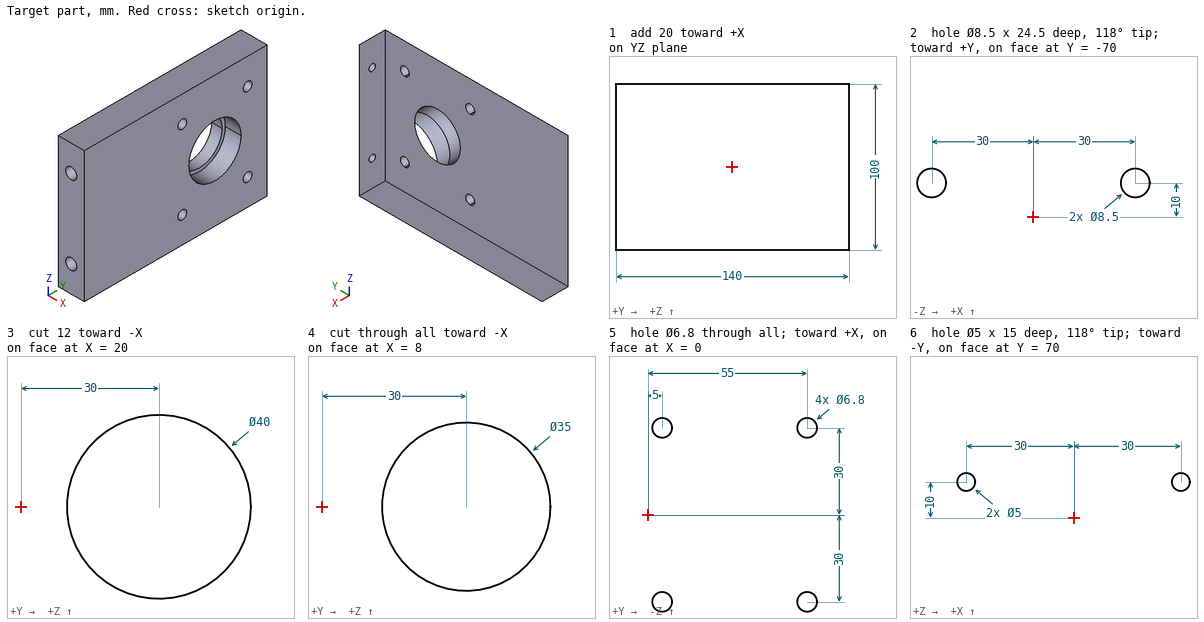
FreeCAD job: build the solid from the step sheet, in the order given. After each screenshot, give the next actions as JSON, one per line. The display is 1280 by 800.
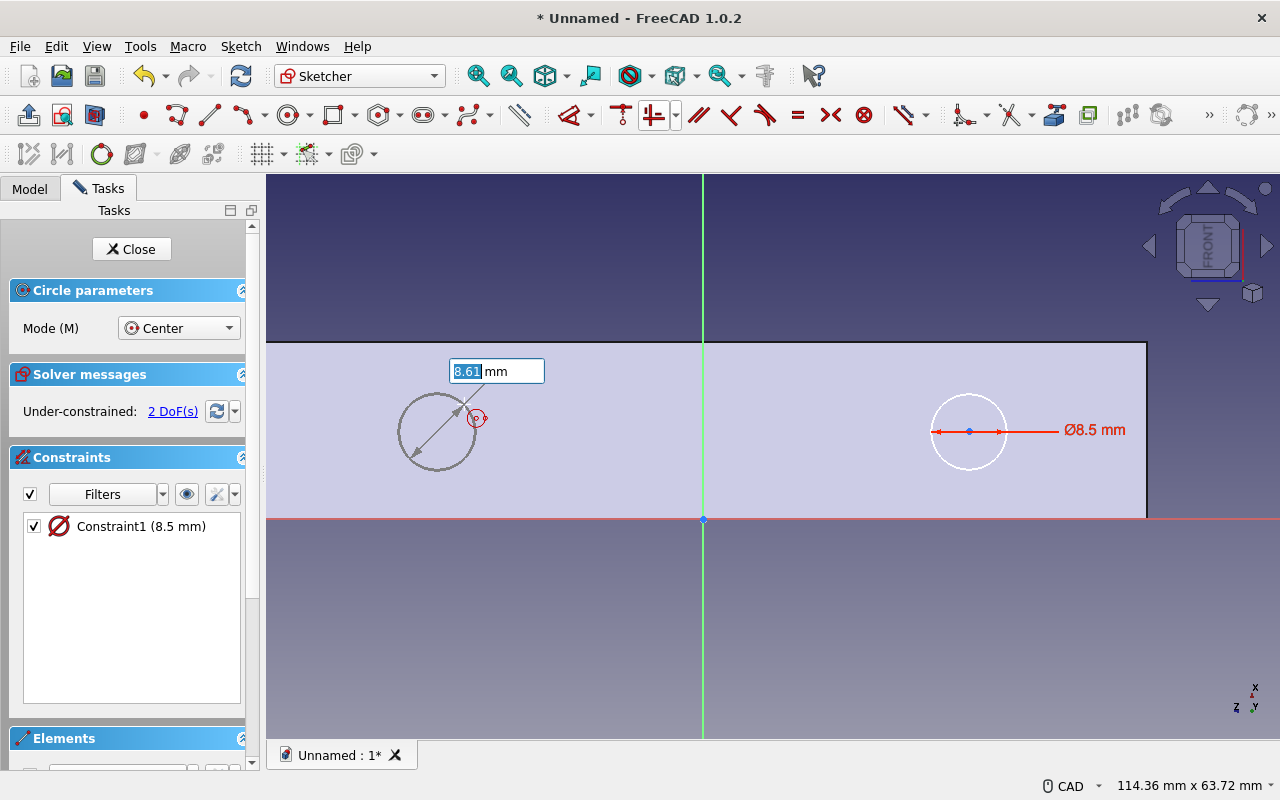
{"action": "type", "text": "8.5"}
{"action": "key", "text": "Return"}
{"action": "key", "text": "Escape"}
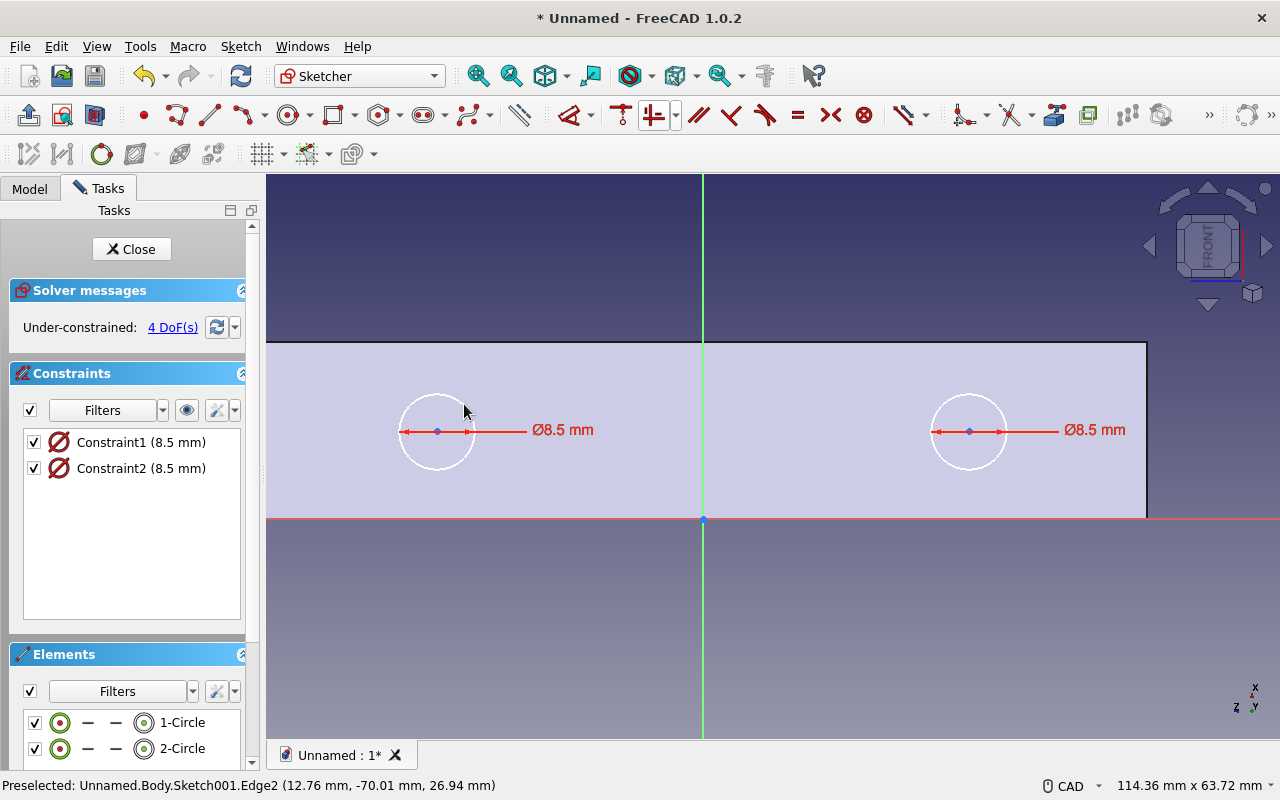
{"action": "left_click", "coordinate": [969, 432]}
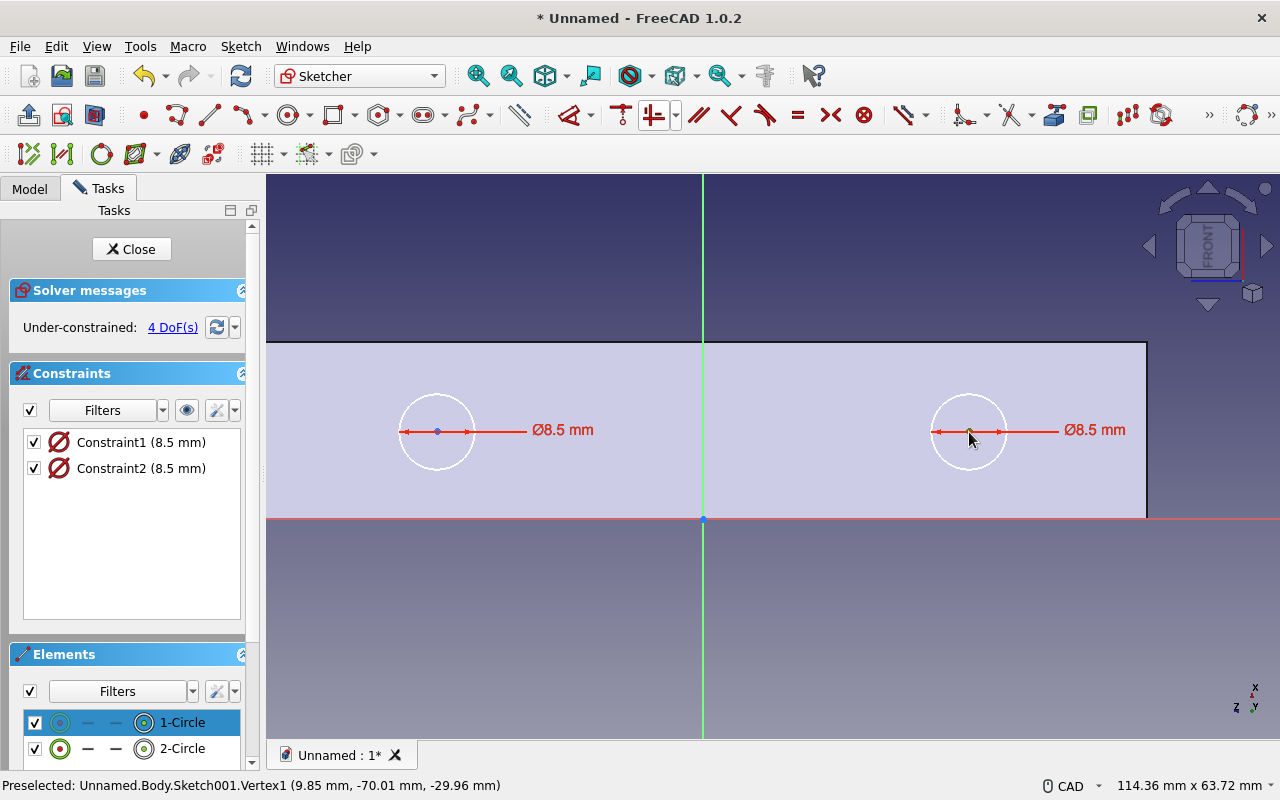
{"action": "left_click", "coordinate": [437, 432]}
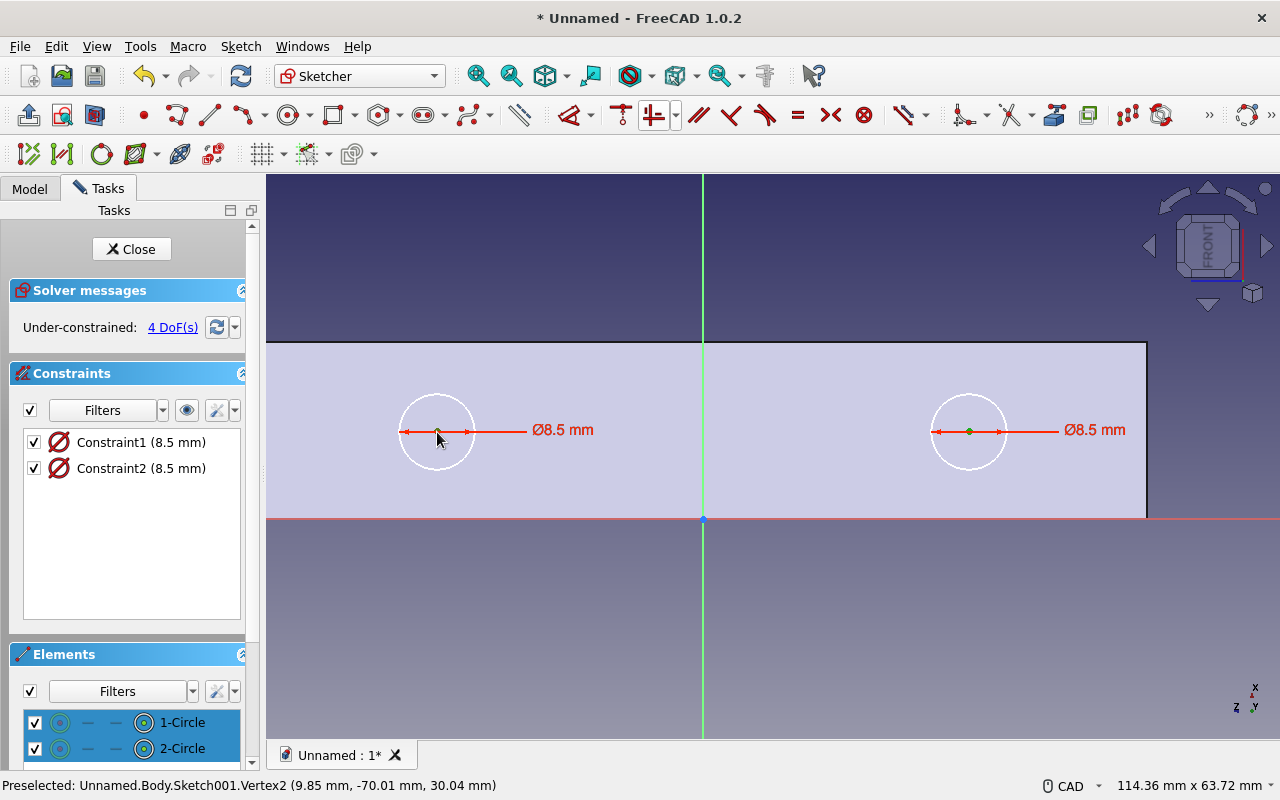
{"action": "left_click", "coordinate": [676, 116]}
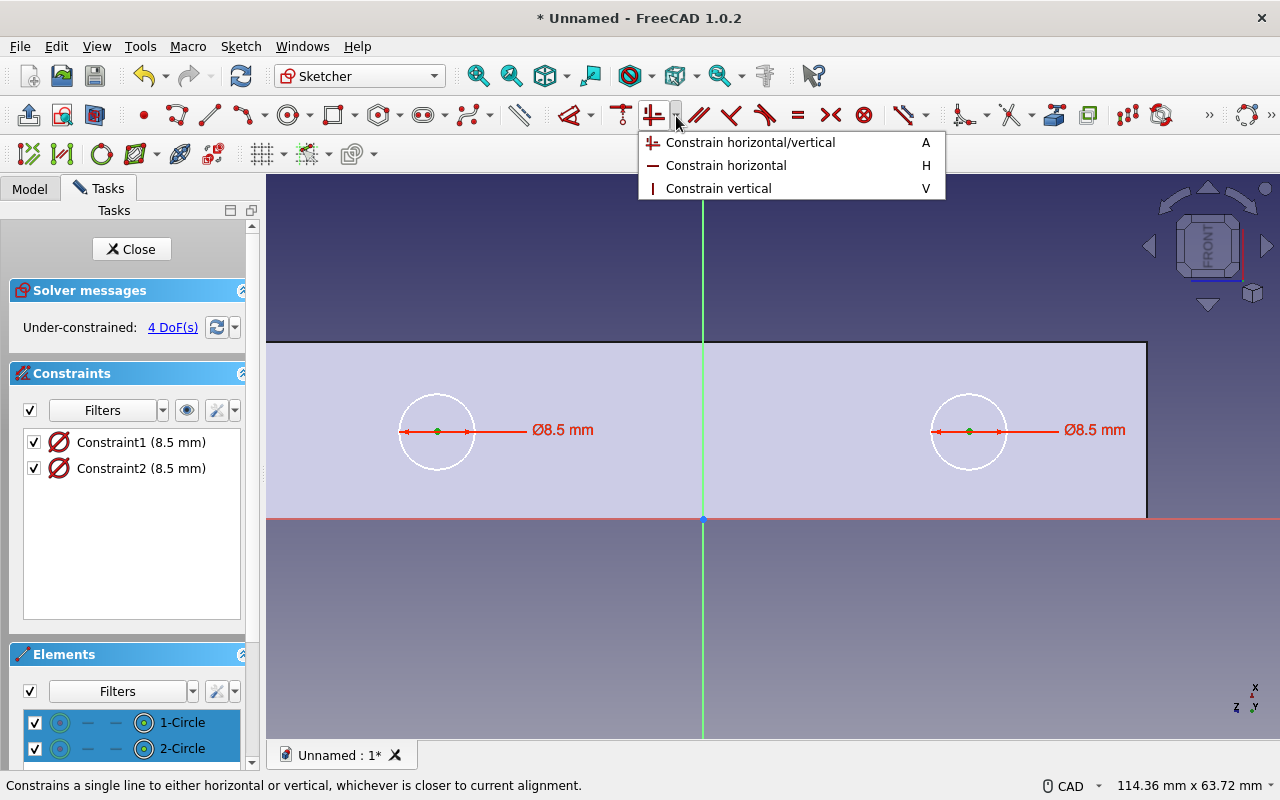
{"action": "left_click", "coordinate": [792, 166]}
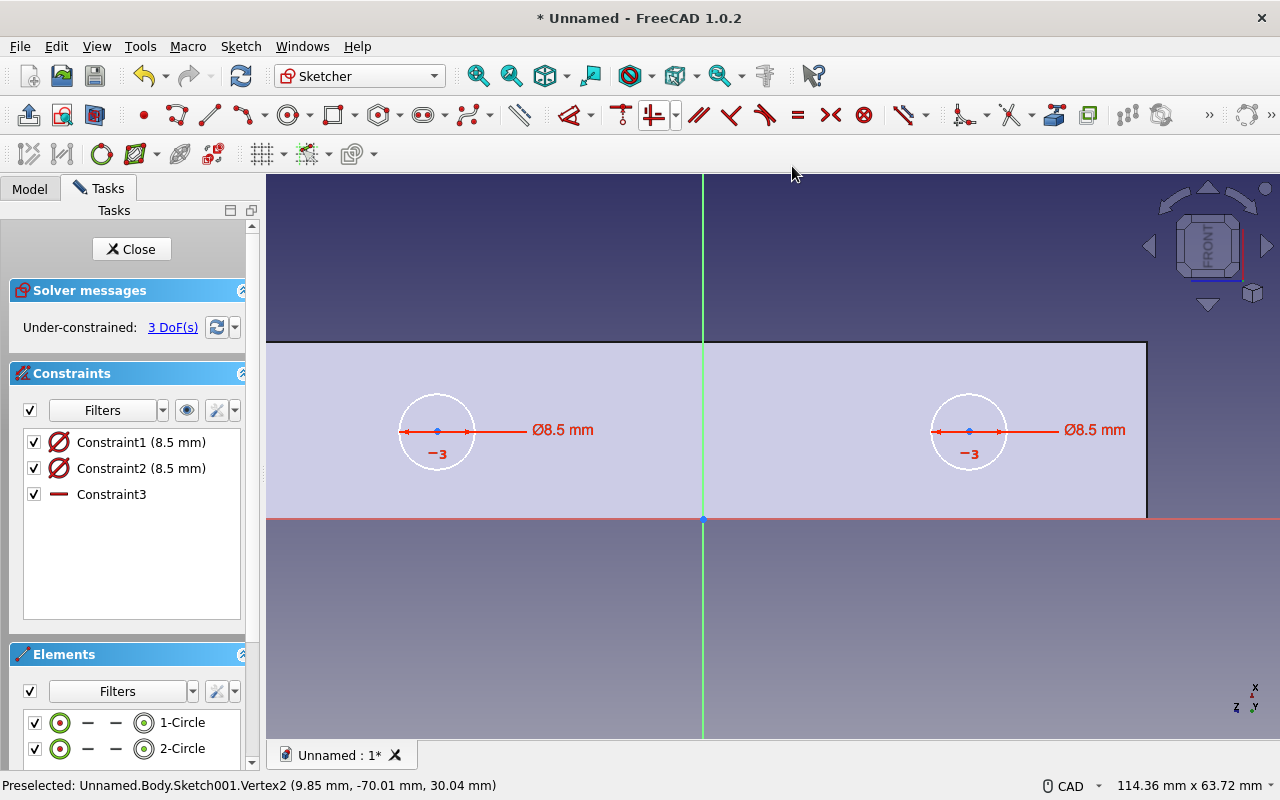
{"action": "left_click", "coordinate": [969, 432]}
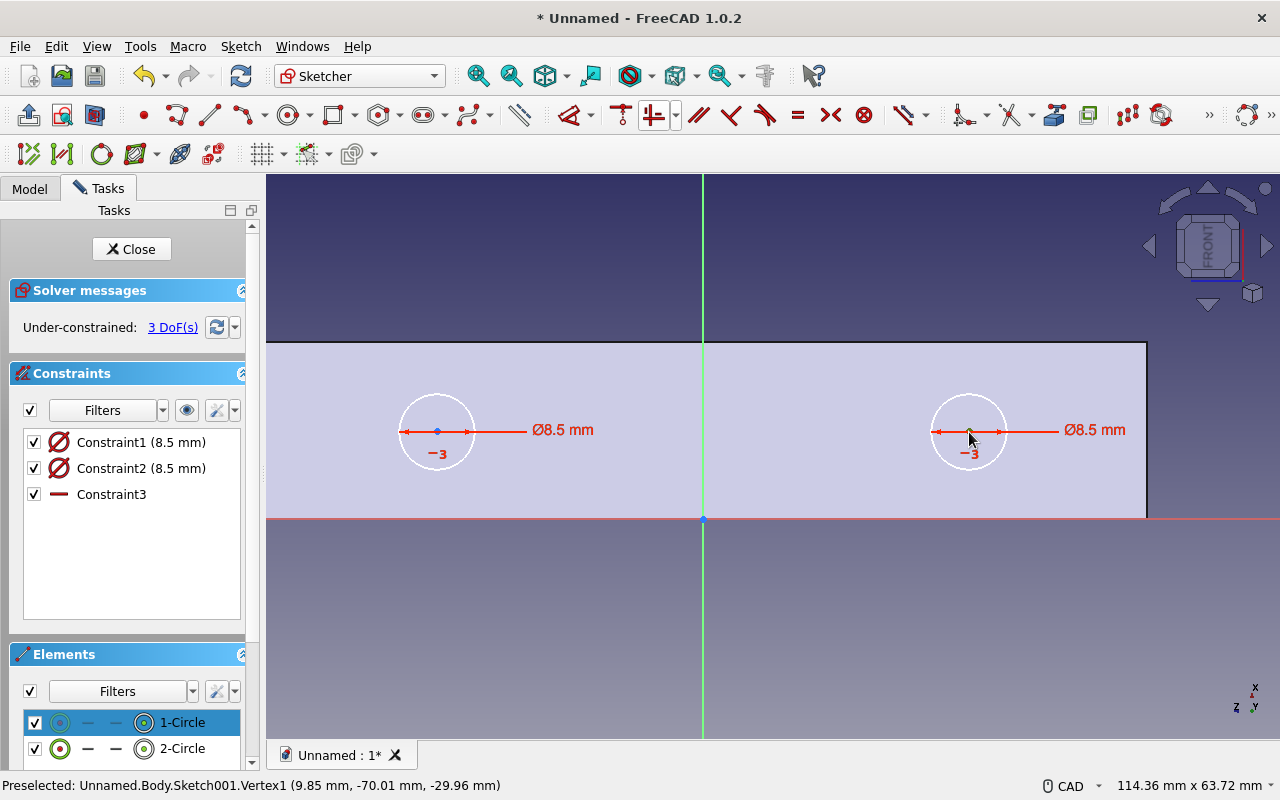
{"action": "left_click", "coordinate": [590, 116]}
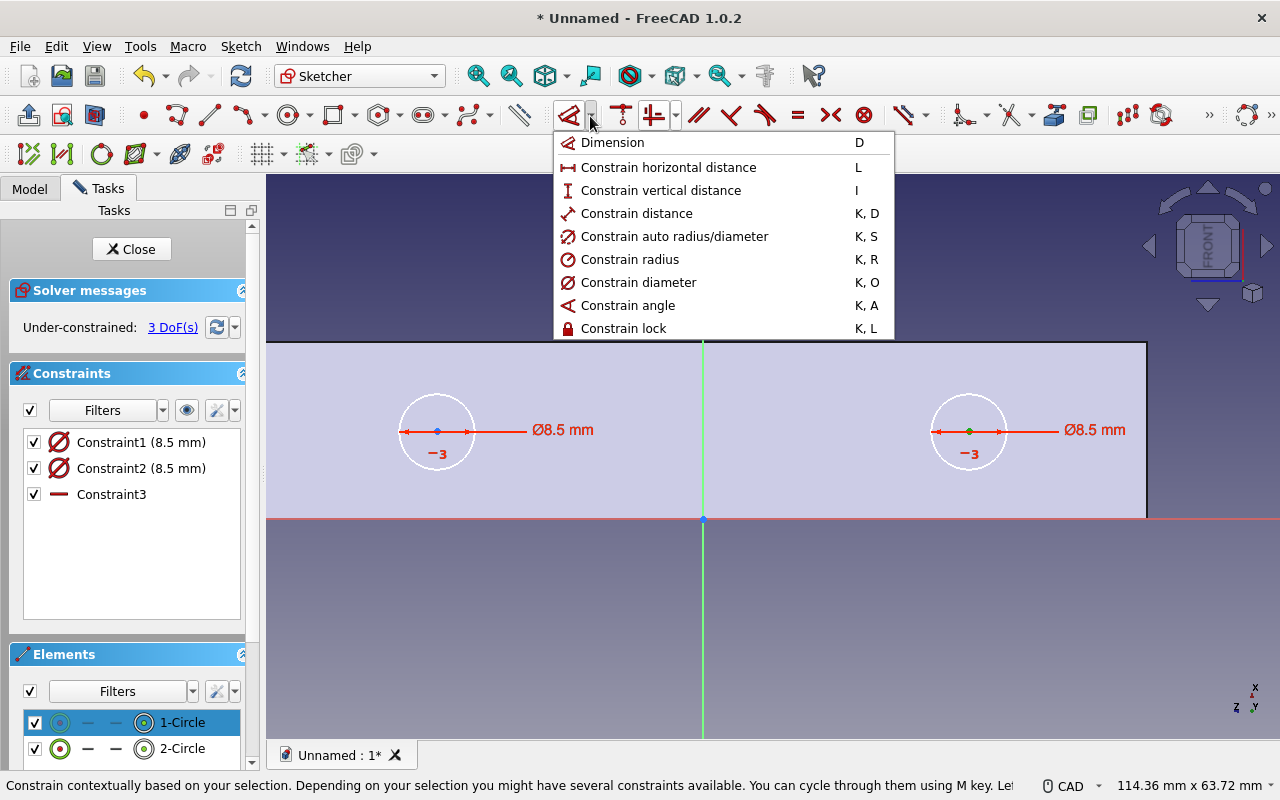
{"action": "left_click", "coordinate": [724, 168]}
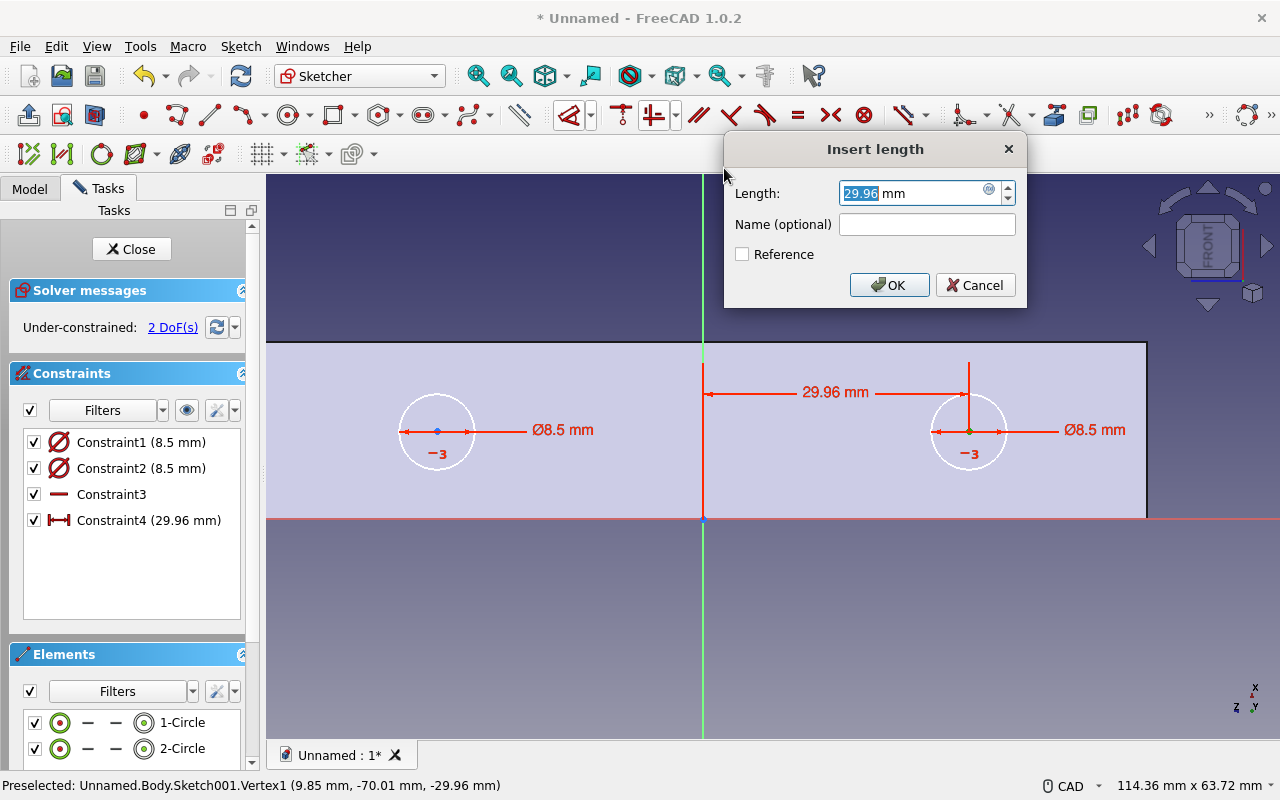
{"action": "type", "text": "30"}
{"action": "key", "text": "Return"}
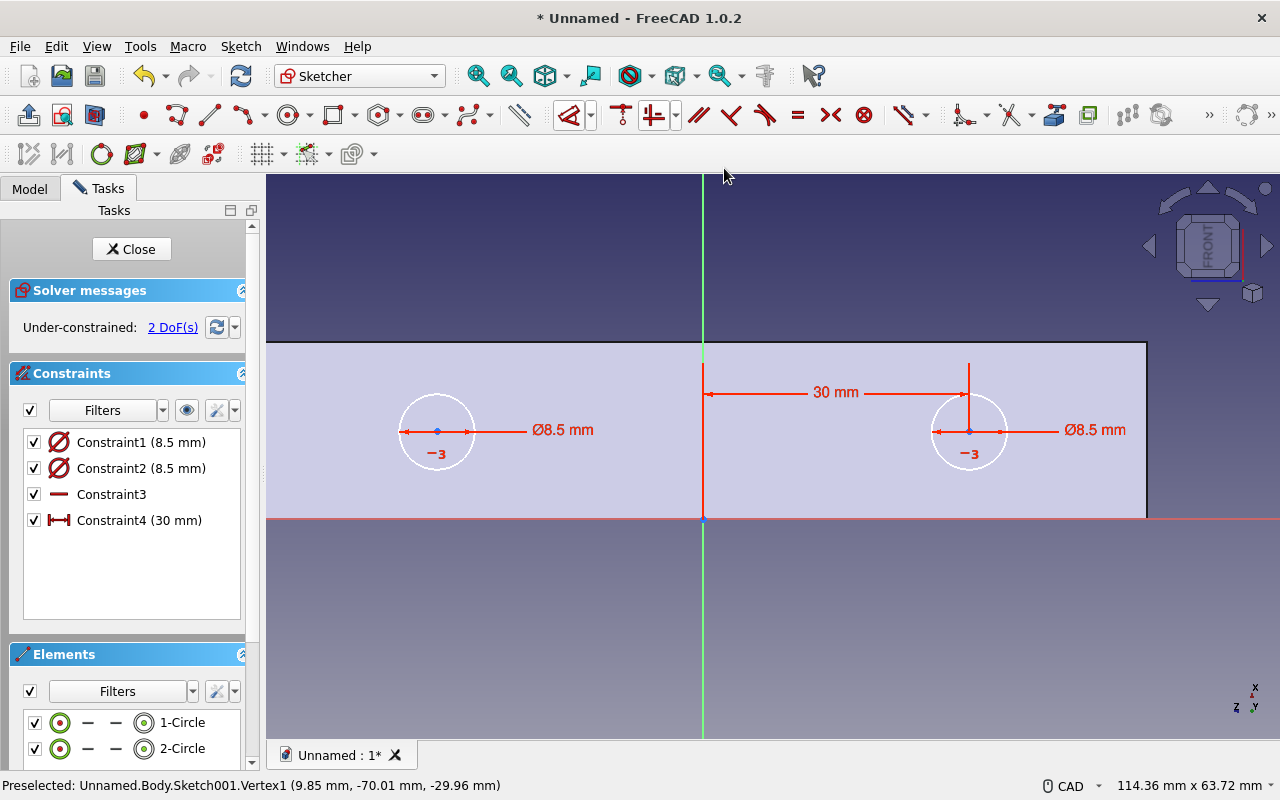
{"action": "left_click", "coordinate": [969, 432]}